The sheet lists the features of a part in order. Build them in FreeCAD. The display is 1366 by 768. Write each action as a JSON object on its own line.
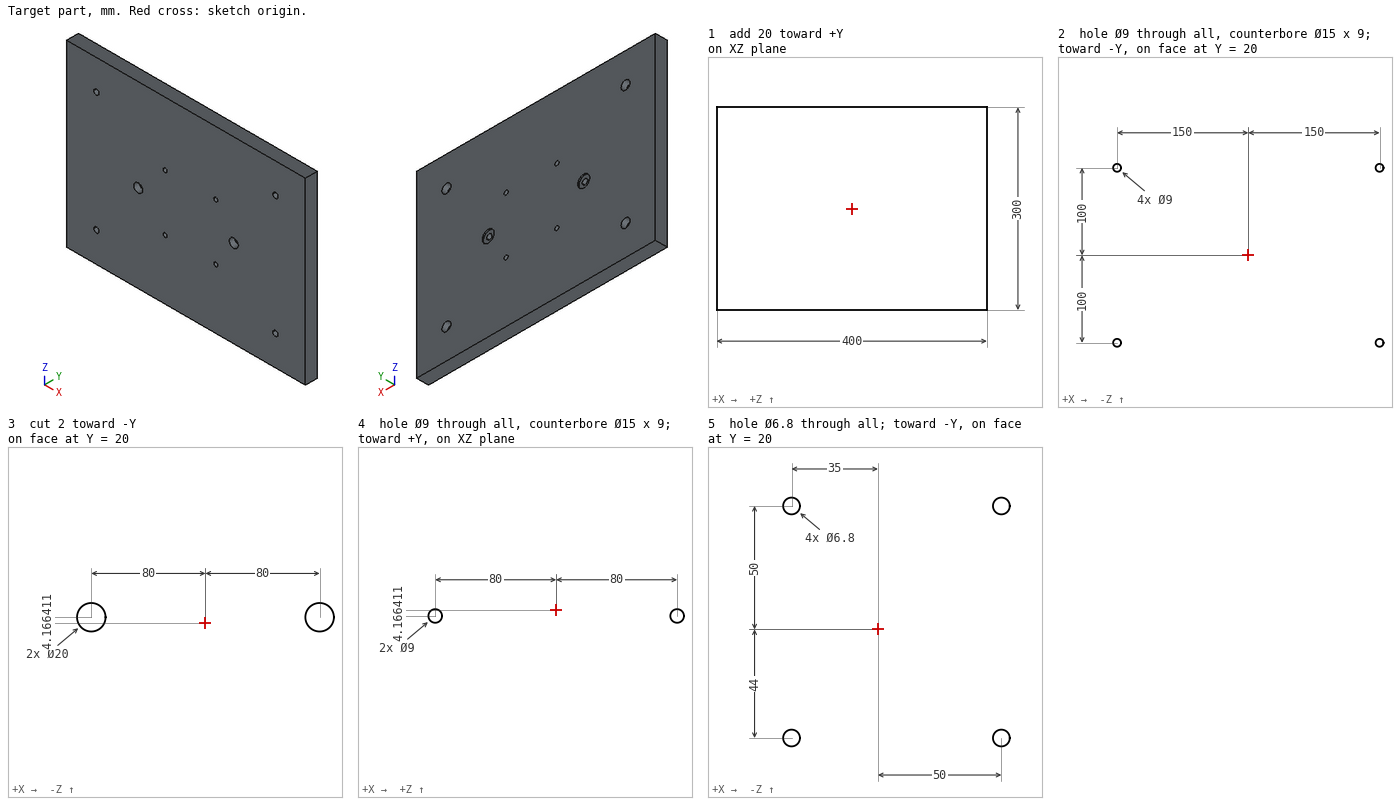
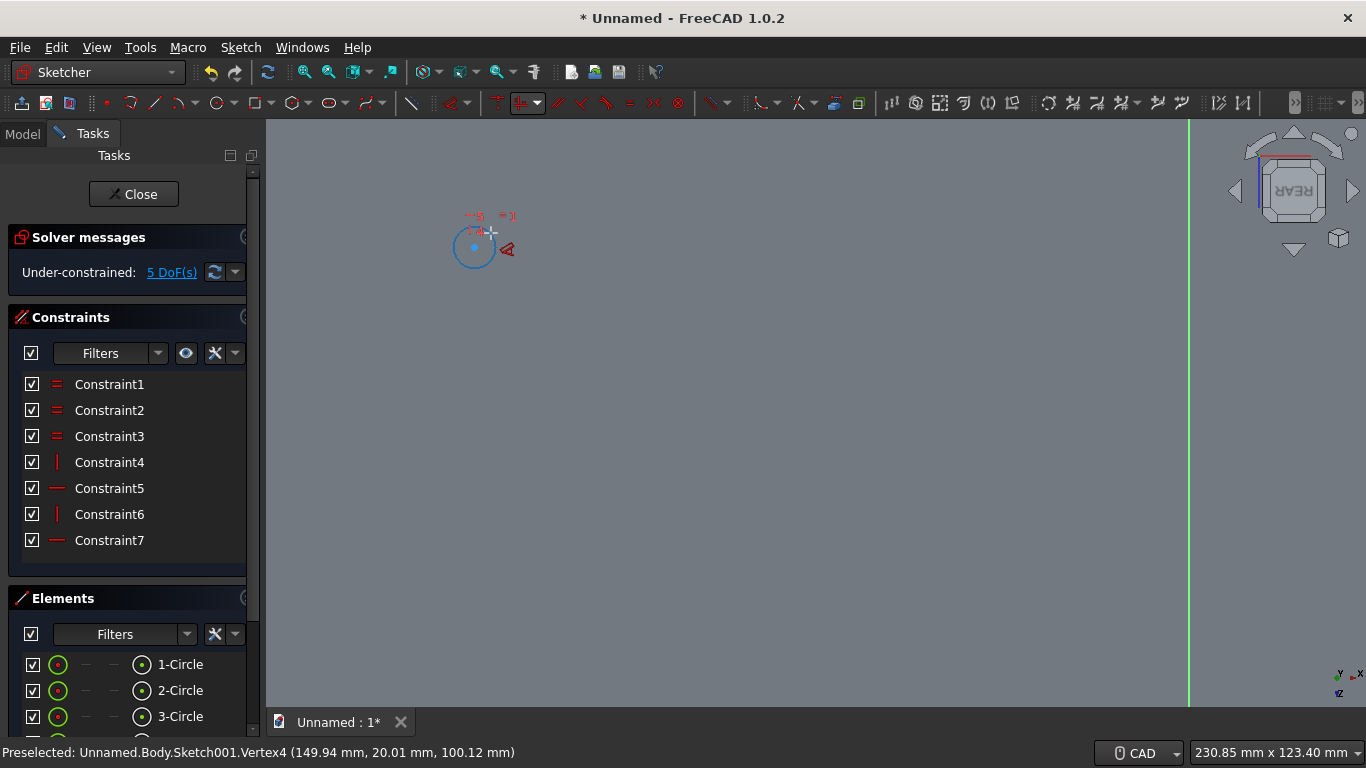
{"action": "left_click", "coordinate": [489, 233]}
{"action": "left_click", "coordinate": [511, 210]}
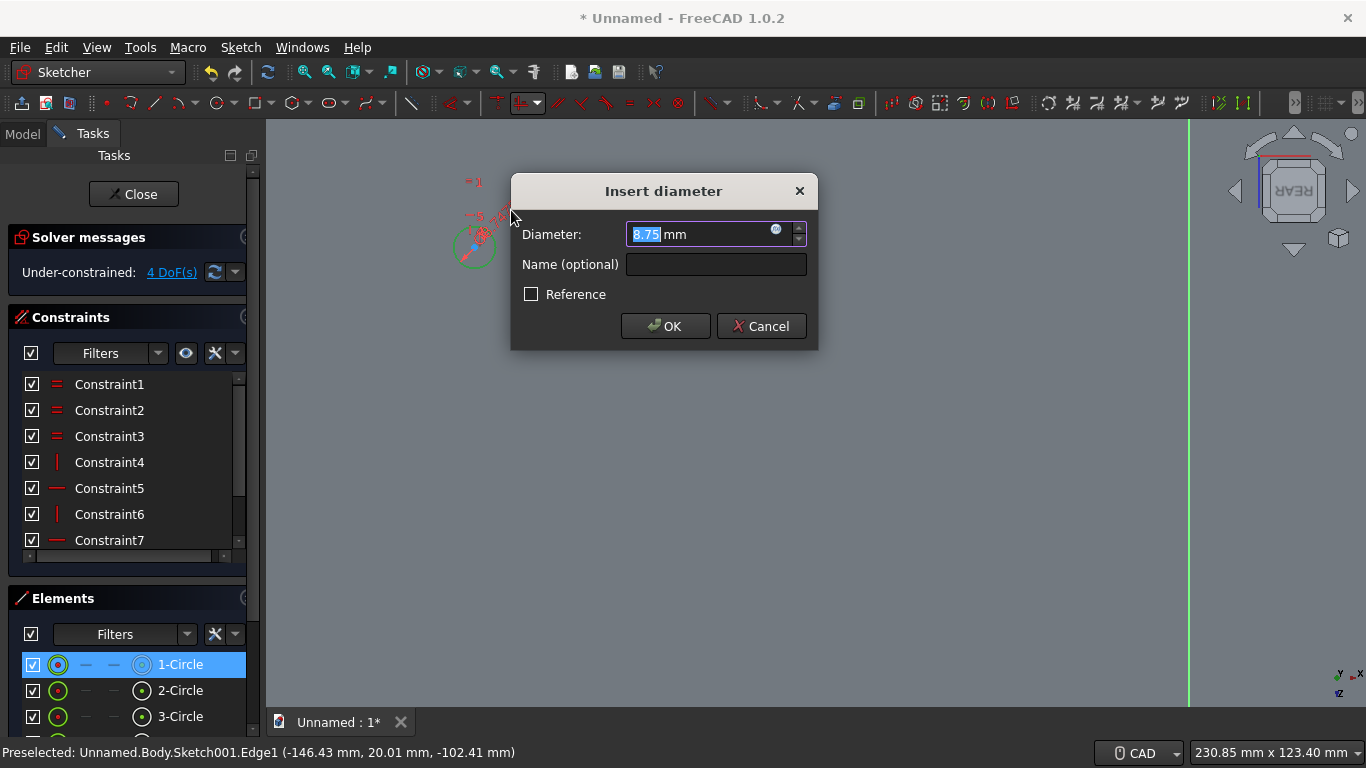
{"action": "type", "text": "9"}
{"action": "key", "text": "Return"}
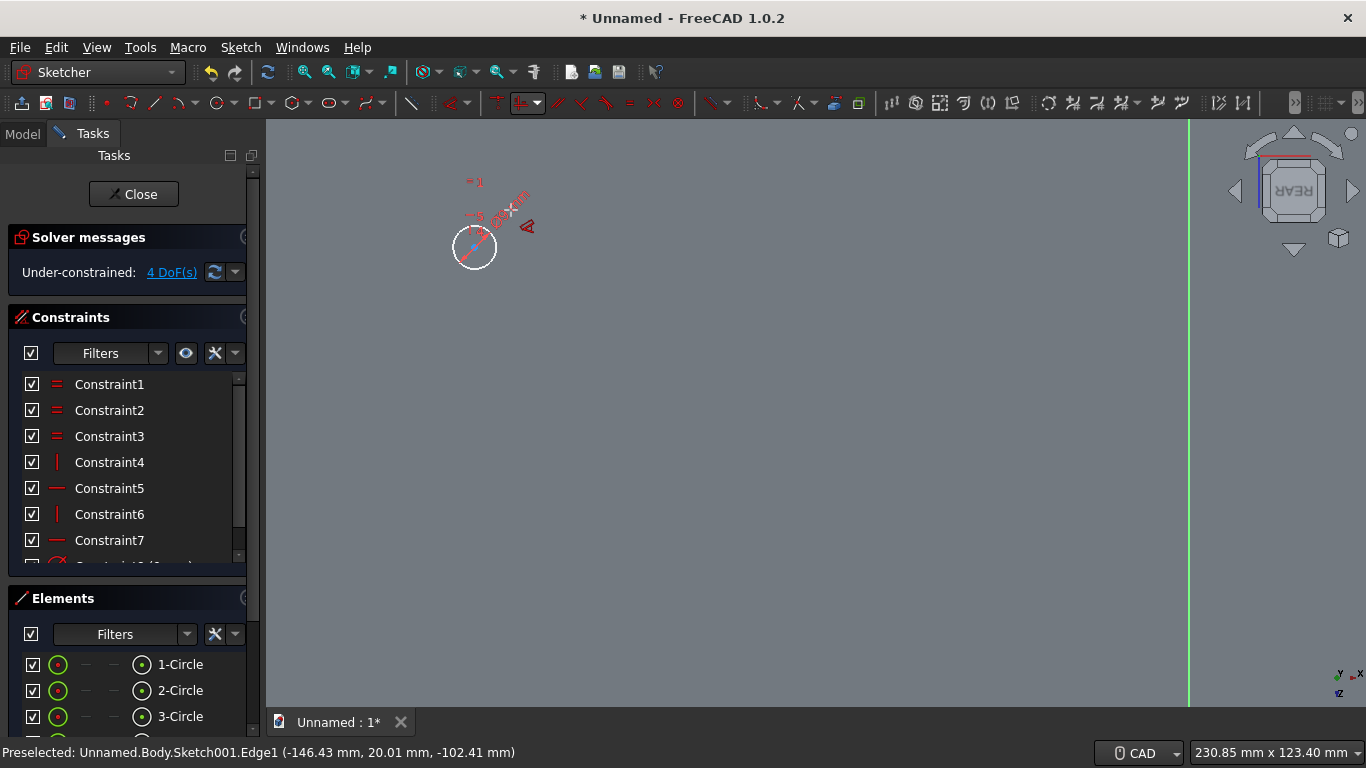
{"action": "left_click", "coordinate": [475, 247]}
{"action": "left_click", "coordinate": [832, 213]}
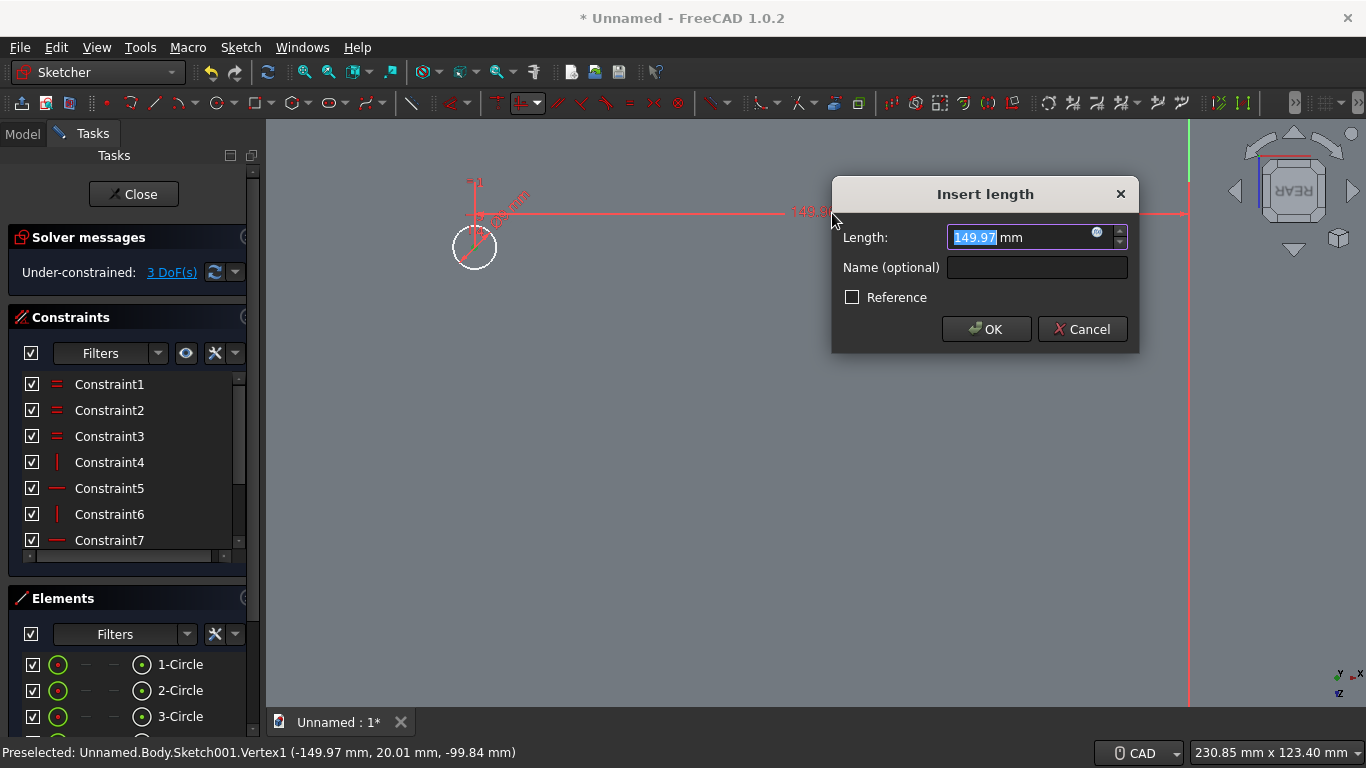
{"action": "type", "text": "150"}
{"action": "key", "text": "Return"}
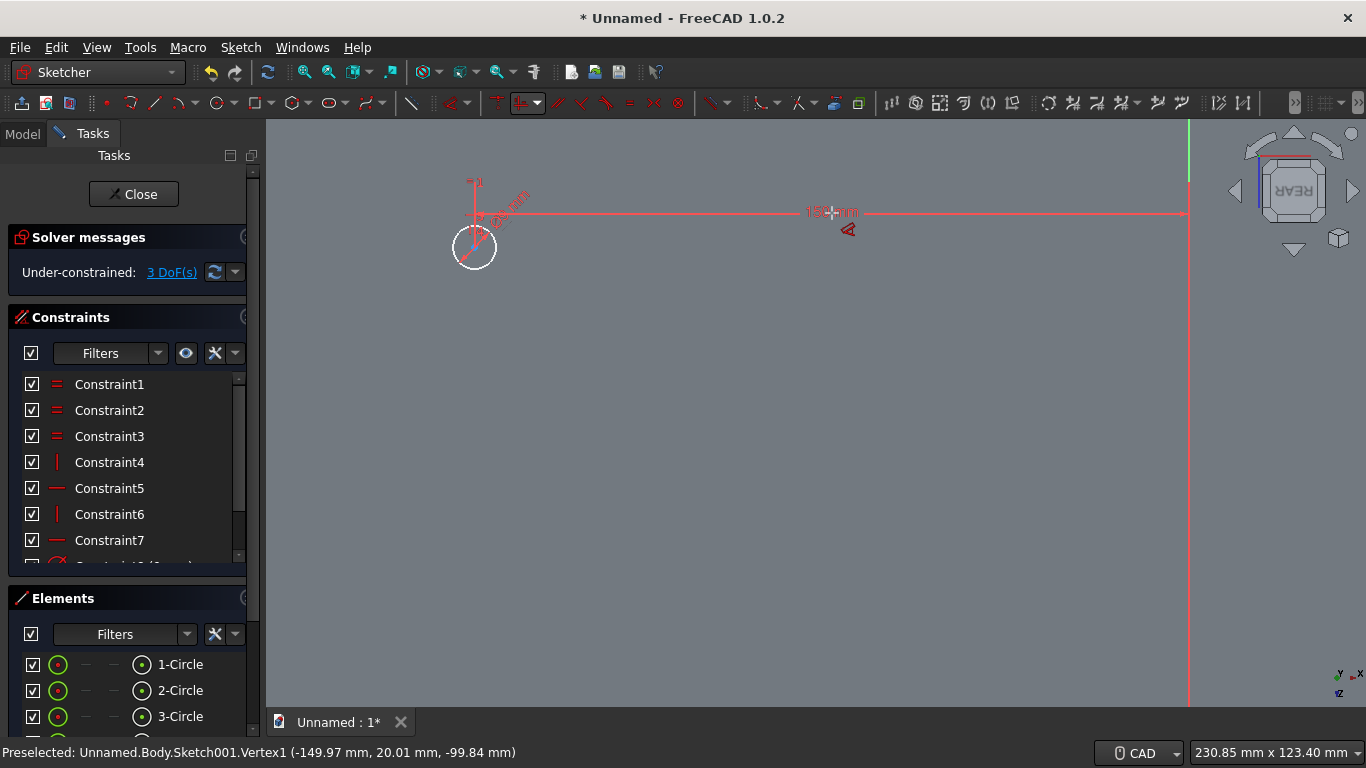
{"action": "left_click", "coordinate": [475, 247]}
{"action": "left_click", "coordinate": [441, 463]}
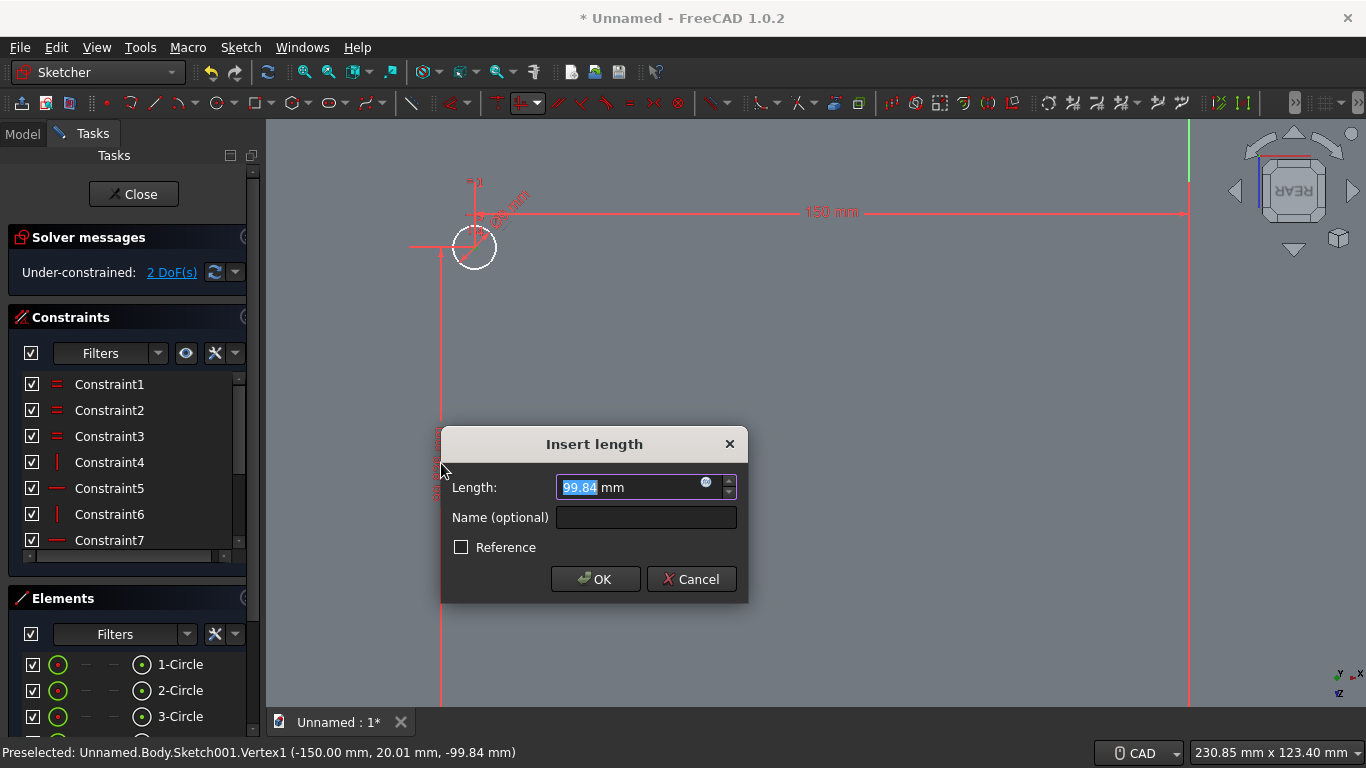
{"action": "type", "text": "100"}
{"action": "key", "text": "Return"}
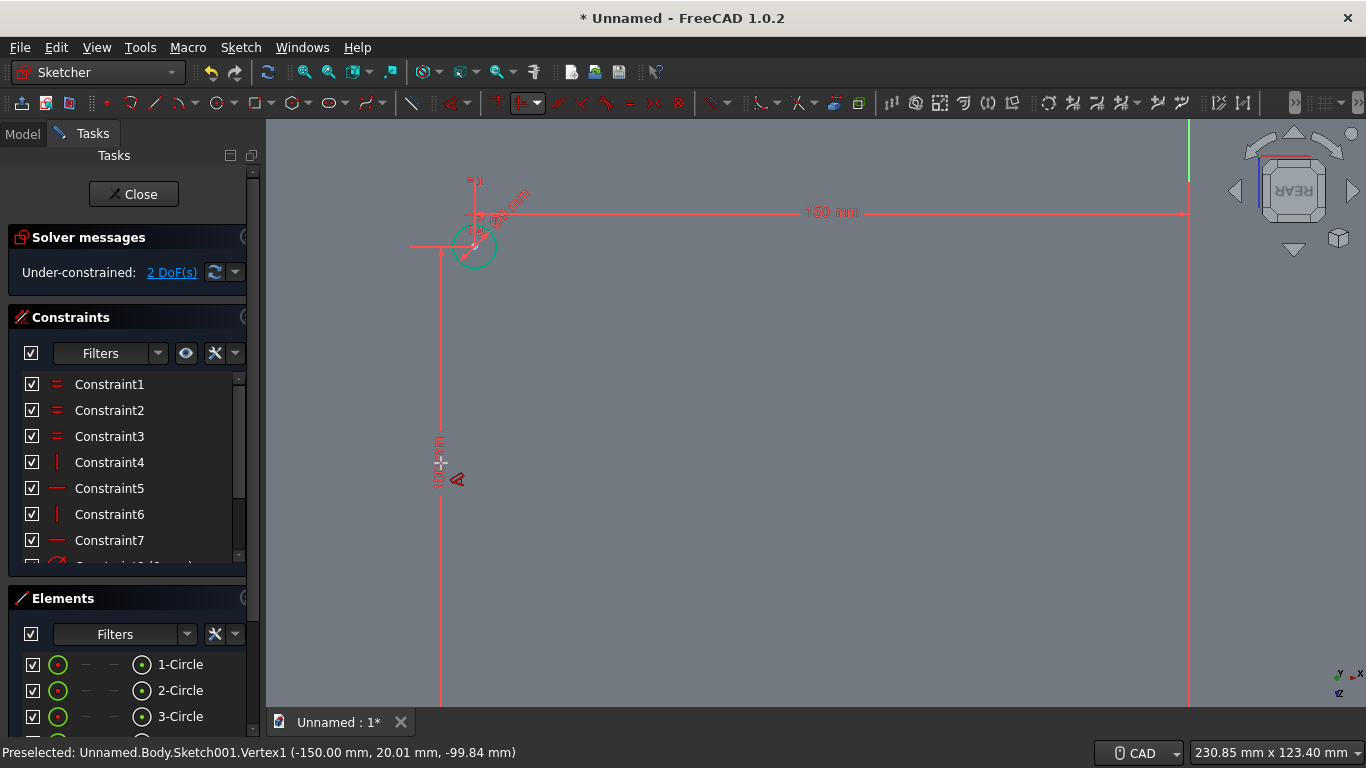
{"action": "scroll", "coordinate": [490, 232], "scroll_direction": "down", "scroll_amount": 5}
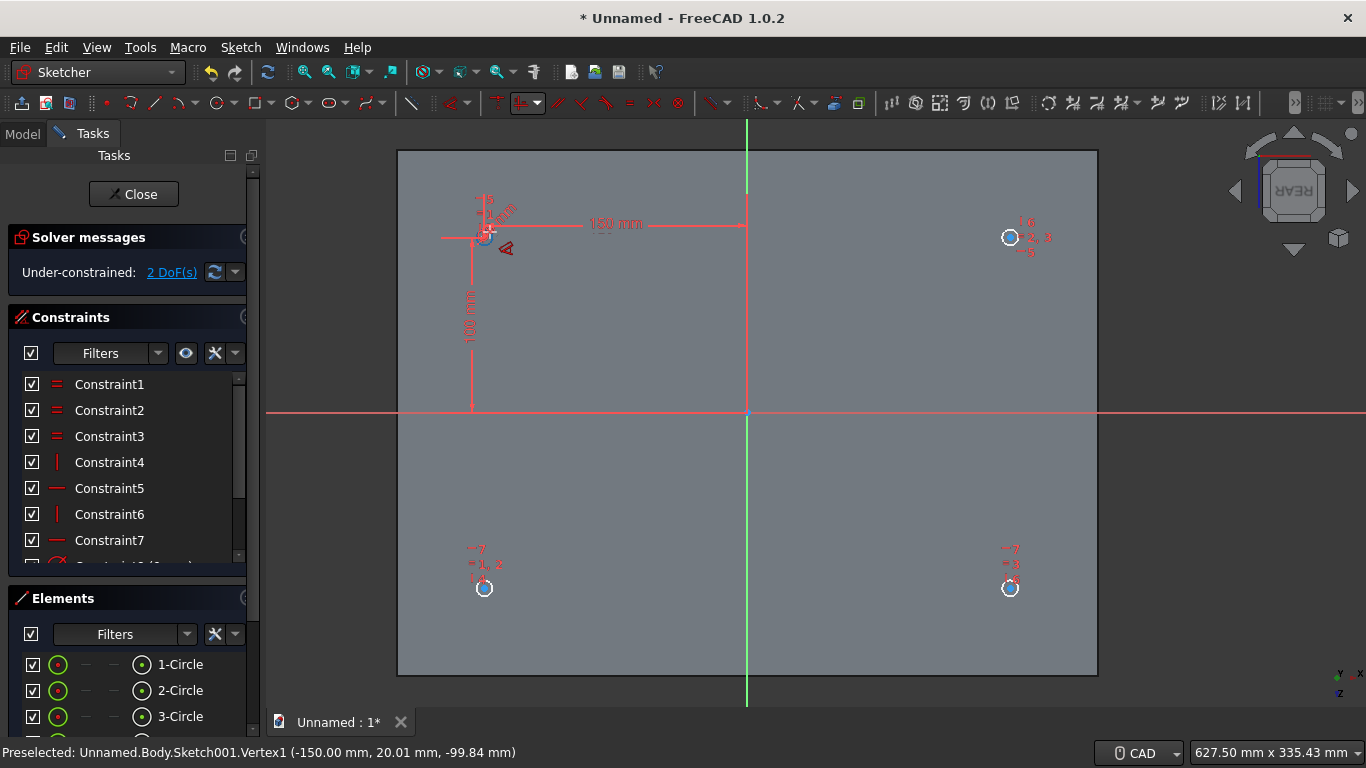
{"action": "left_click", "coordinate": [484, 588]}
{"action": "left_click", "coordinate": [450, 501]}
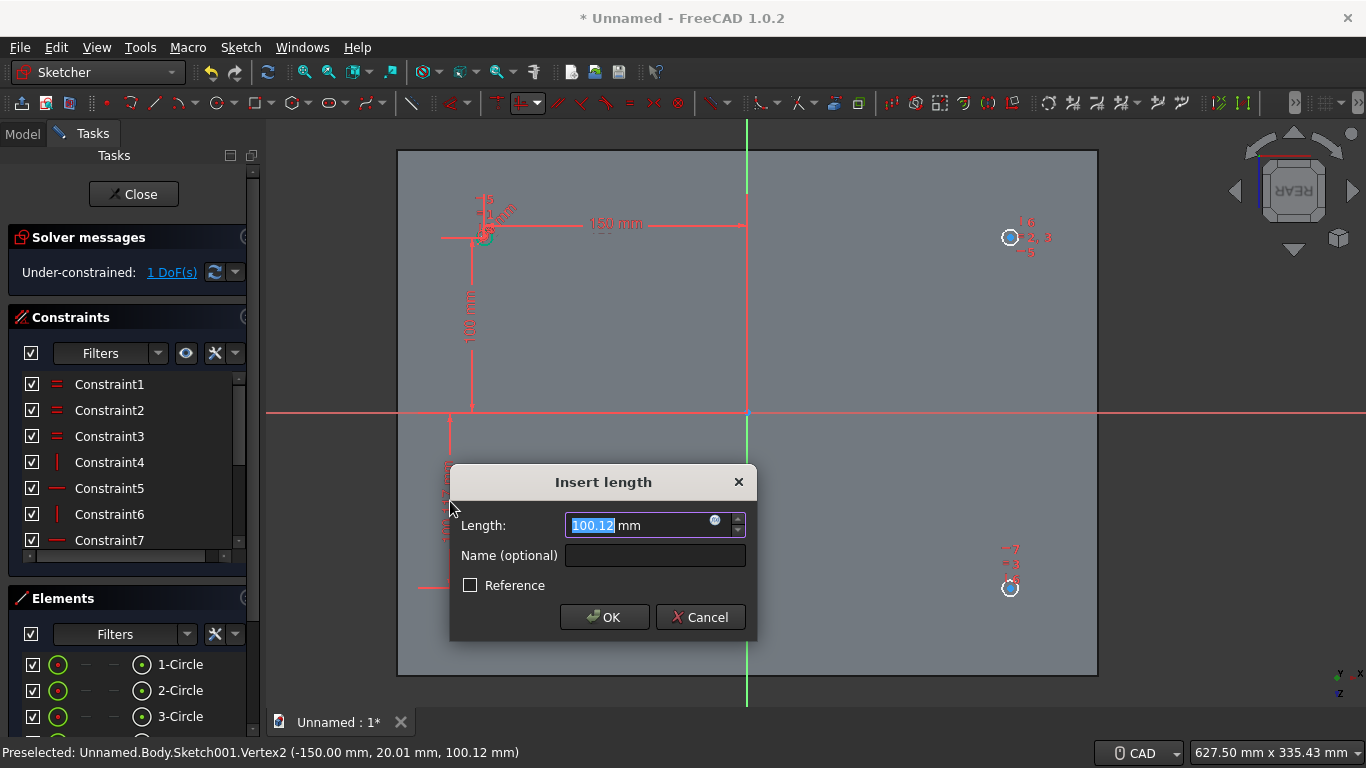
{"action": "type", "text": "100"}
{"action": "key", "text": "Return"}